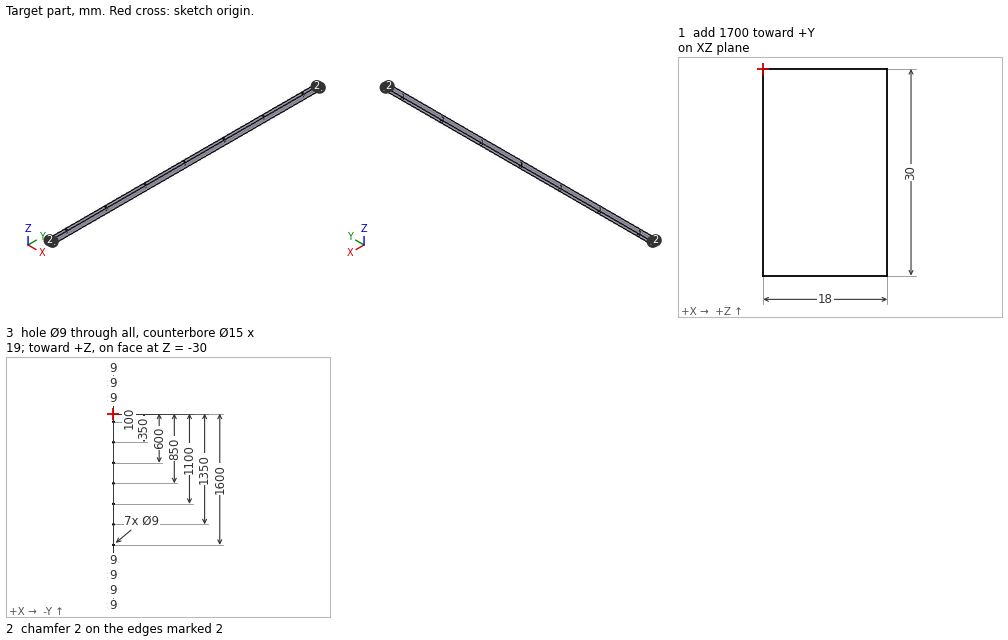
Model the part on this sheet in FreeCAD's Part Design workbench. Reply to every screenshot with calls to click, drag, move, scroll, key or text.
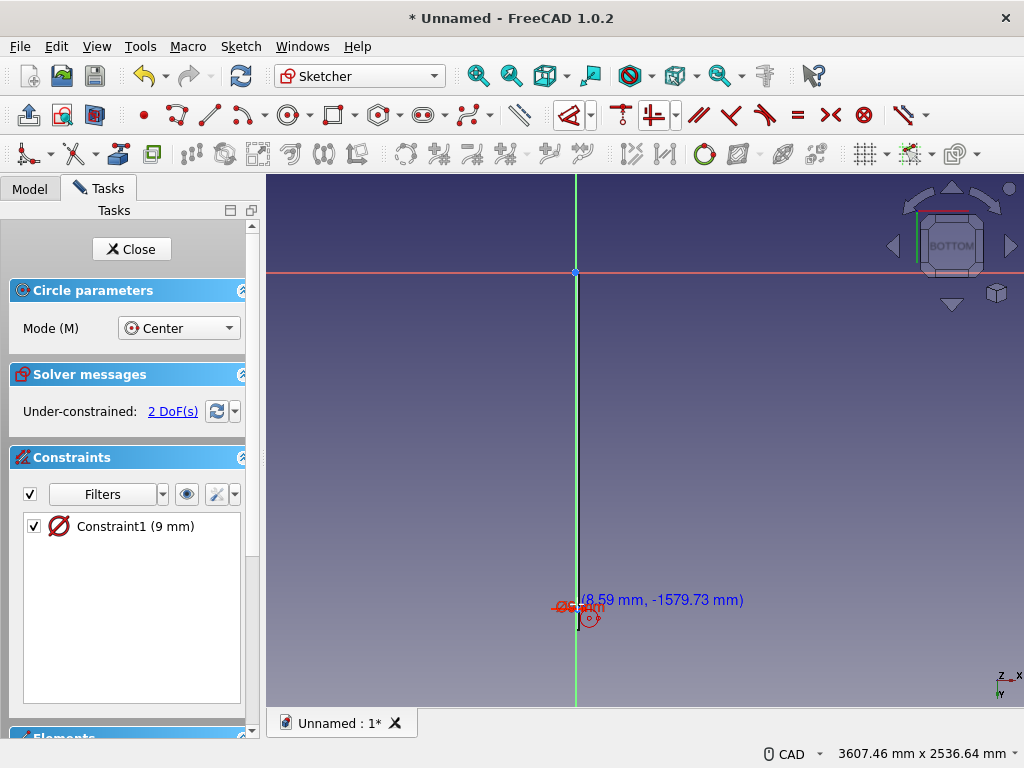
scroll(577, 557, up, 16)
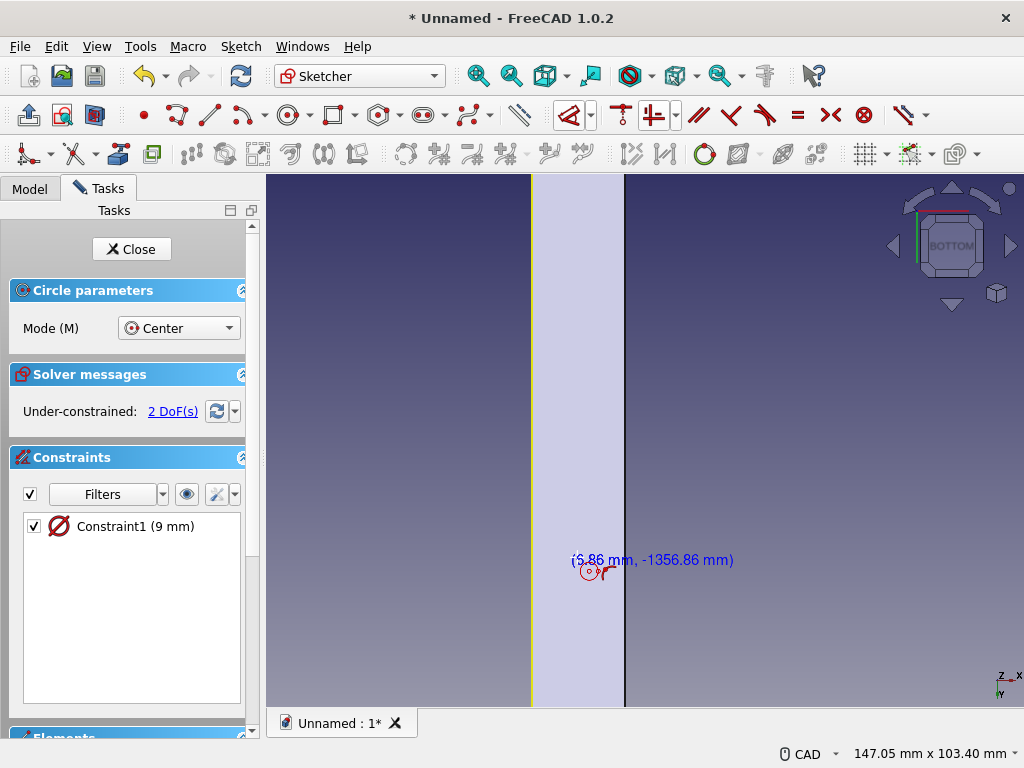
scroll(577, 584, down, 15)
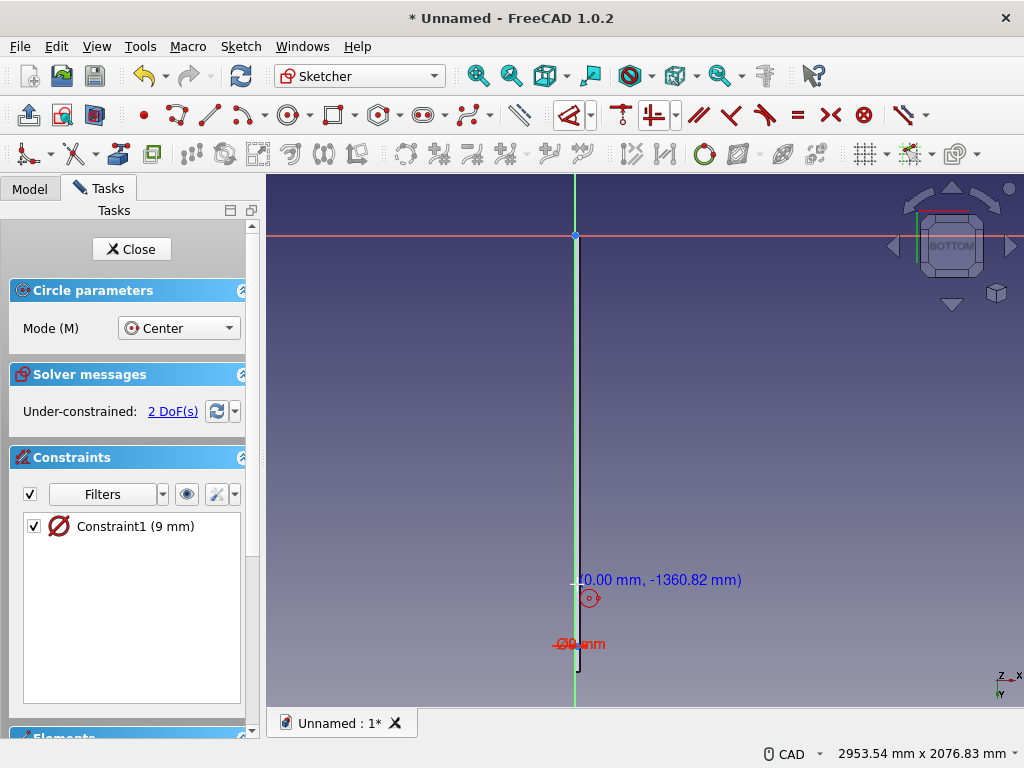
scroll(577, 582, up, 10)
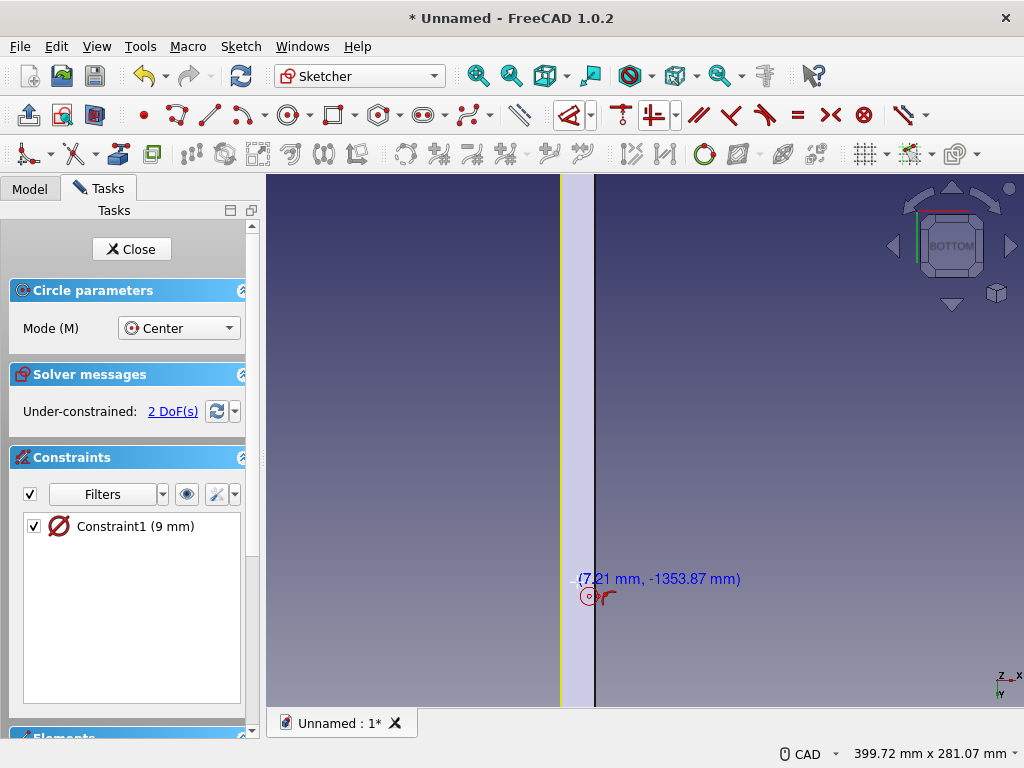
click(578, 577)
move(584, 571)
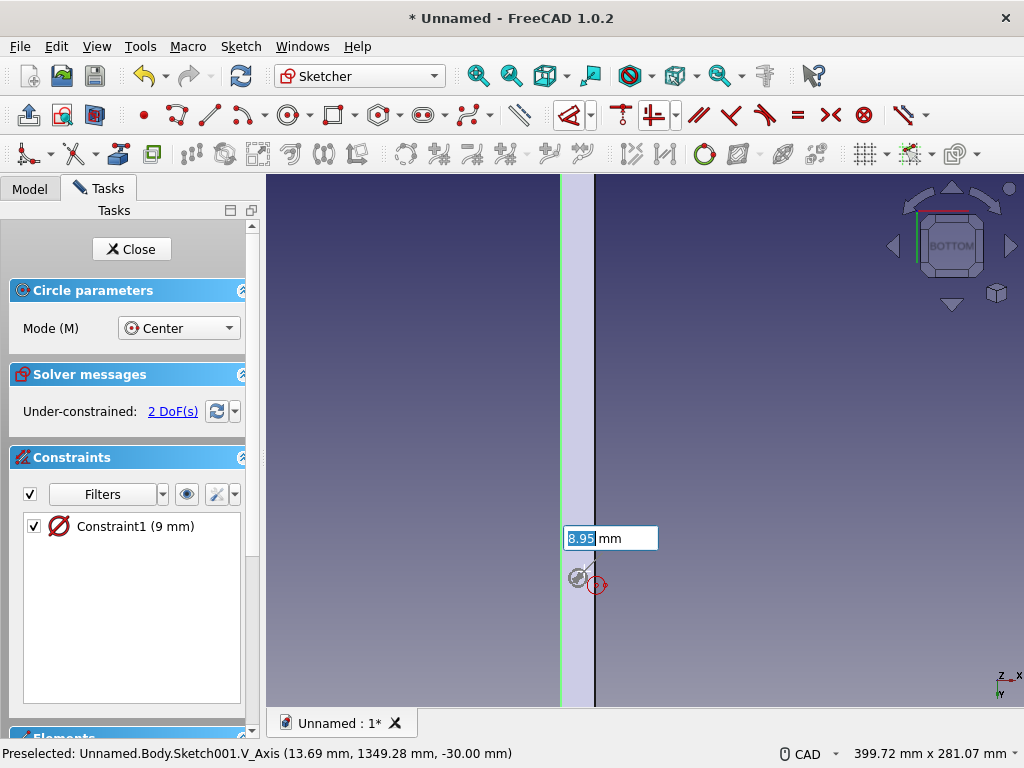
text(9)
key(Return)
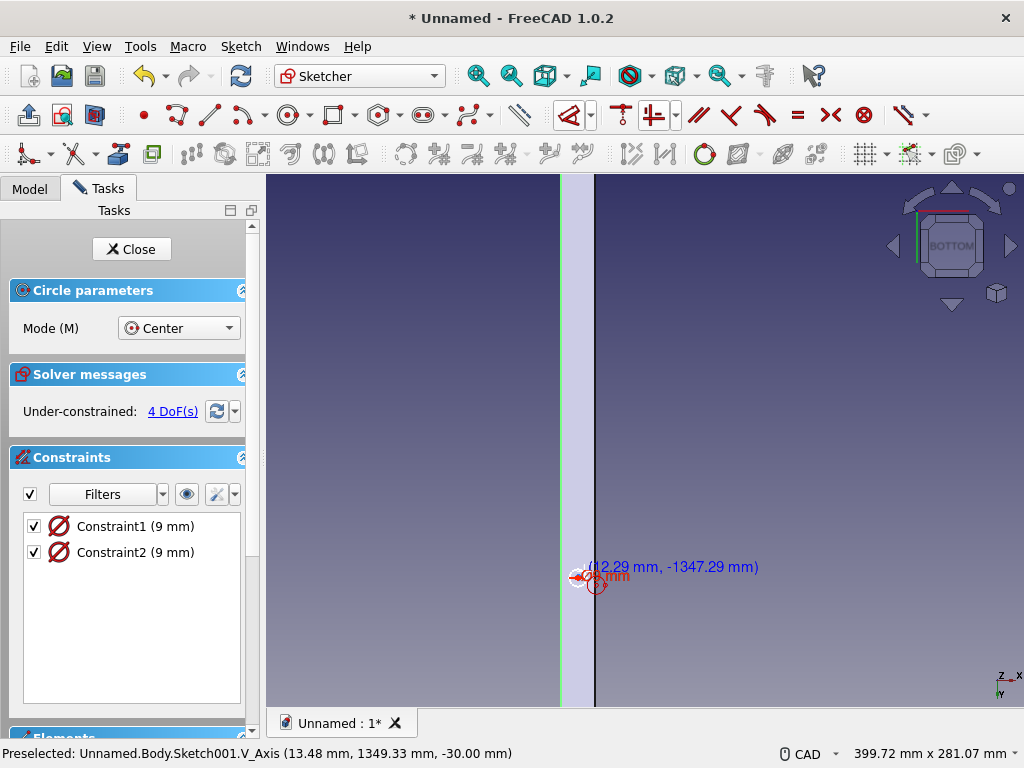
scroll(577, 553, down, 11)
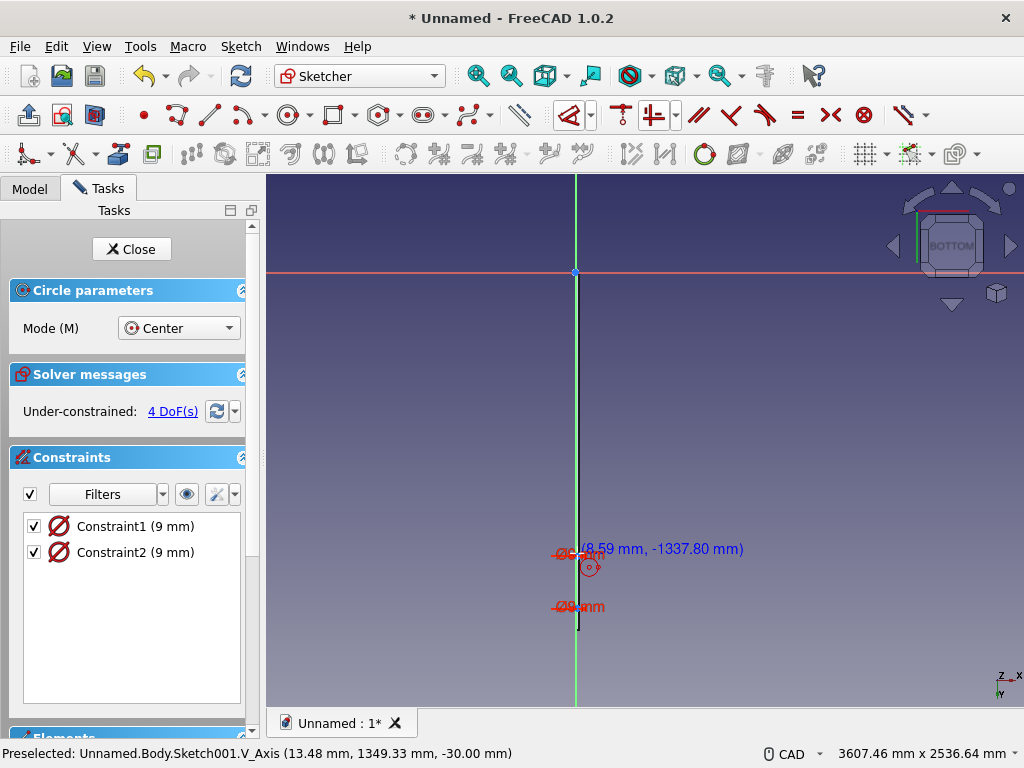
scroll(577, 504, up, 16)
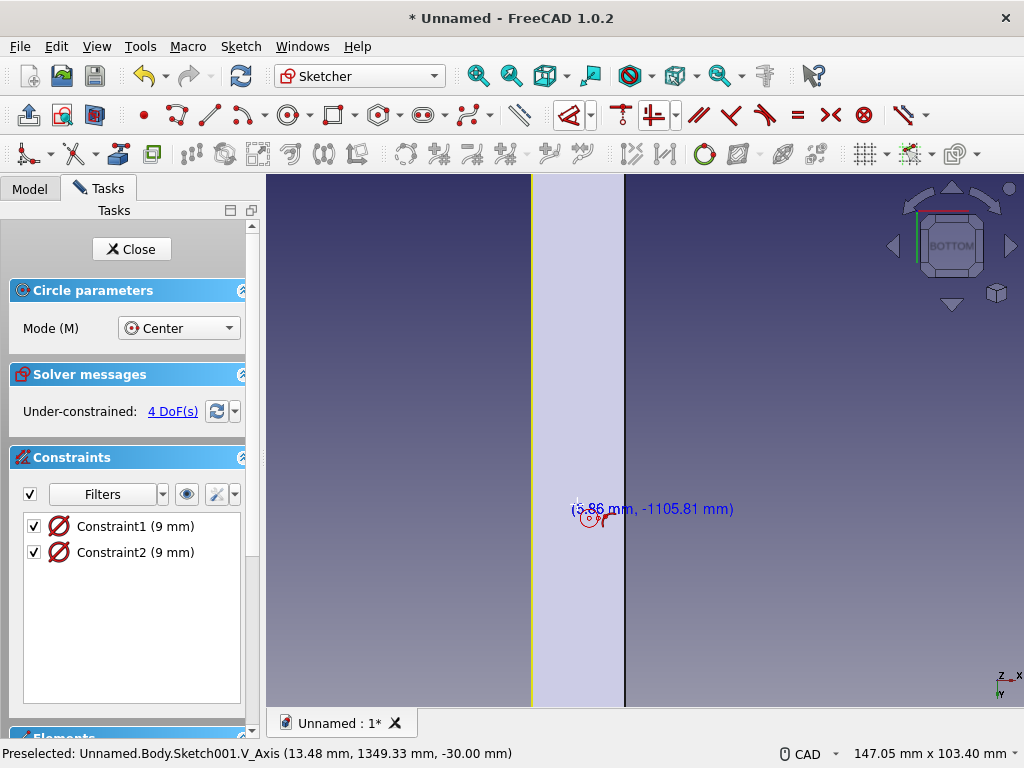
scroll(577, 519, down, 15)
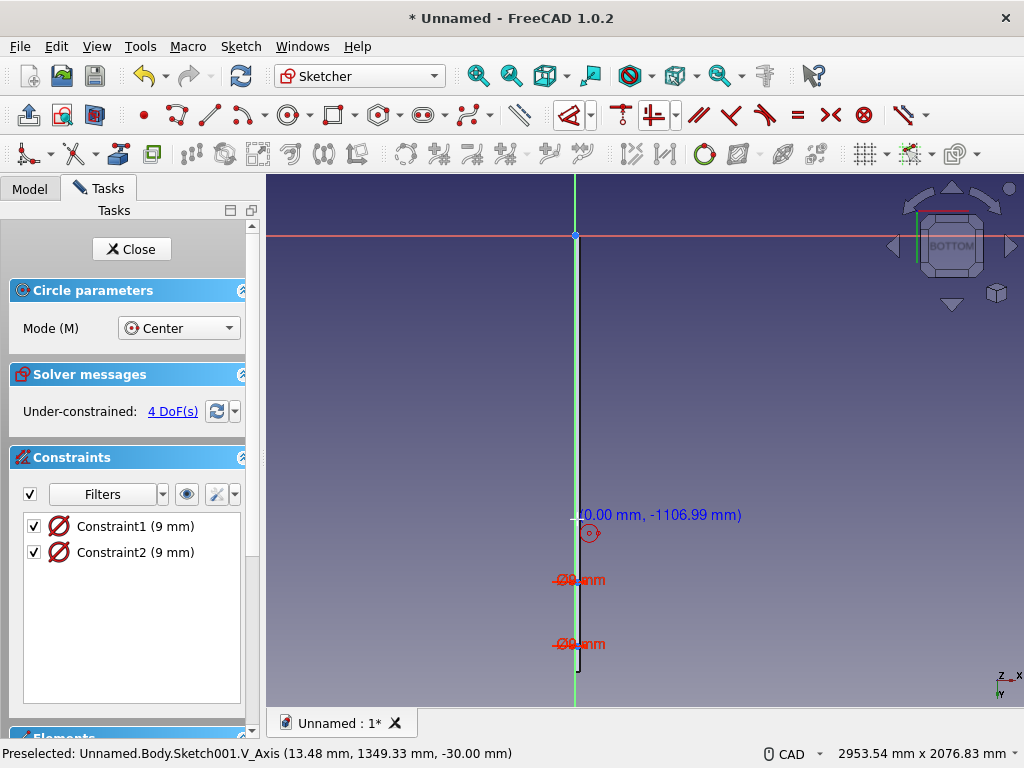
scroll(577, 518, up, 10)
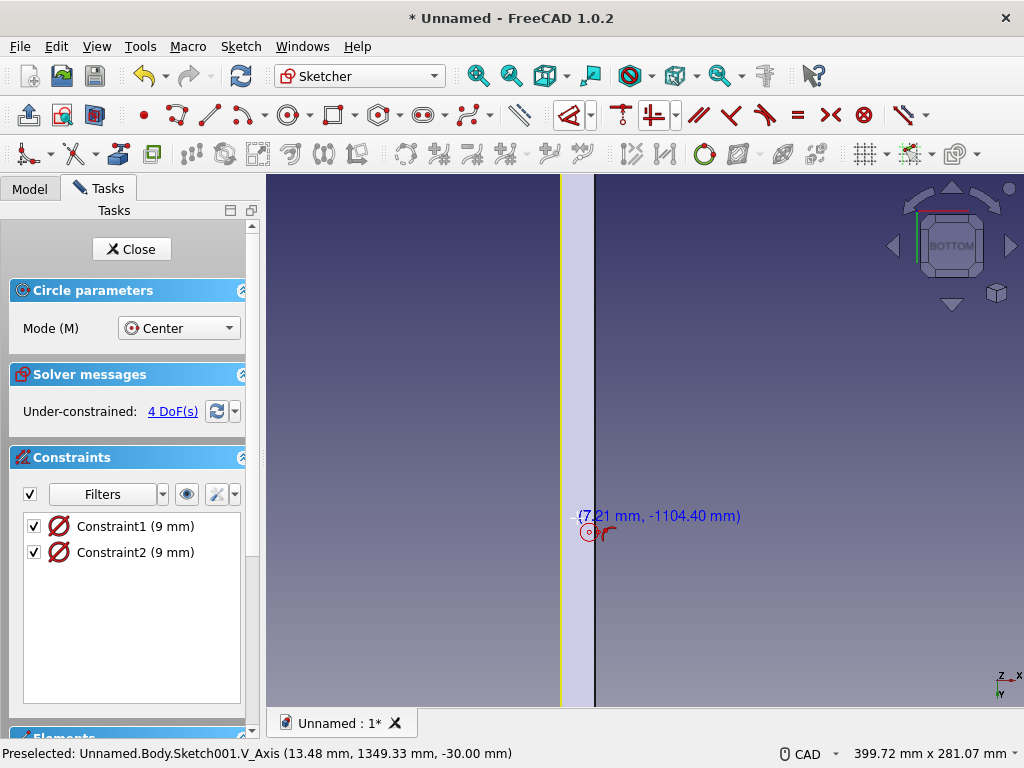
click(578, 513)
move(584, 507)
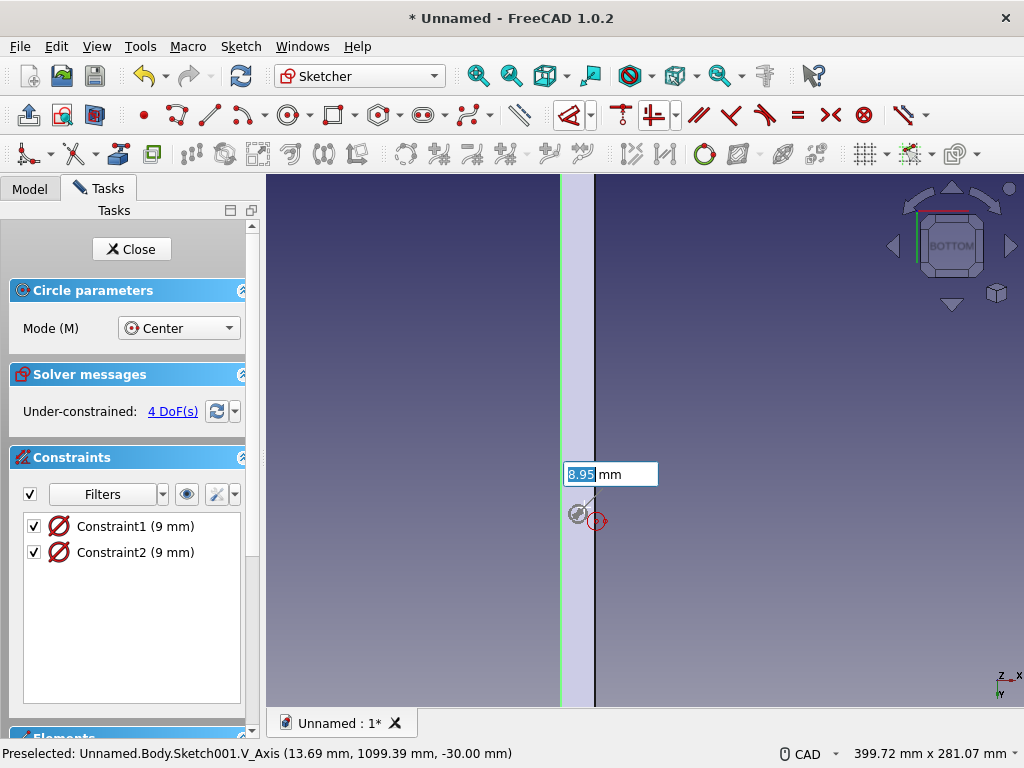
text(9)
key(Return)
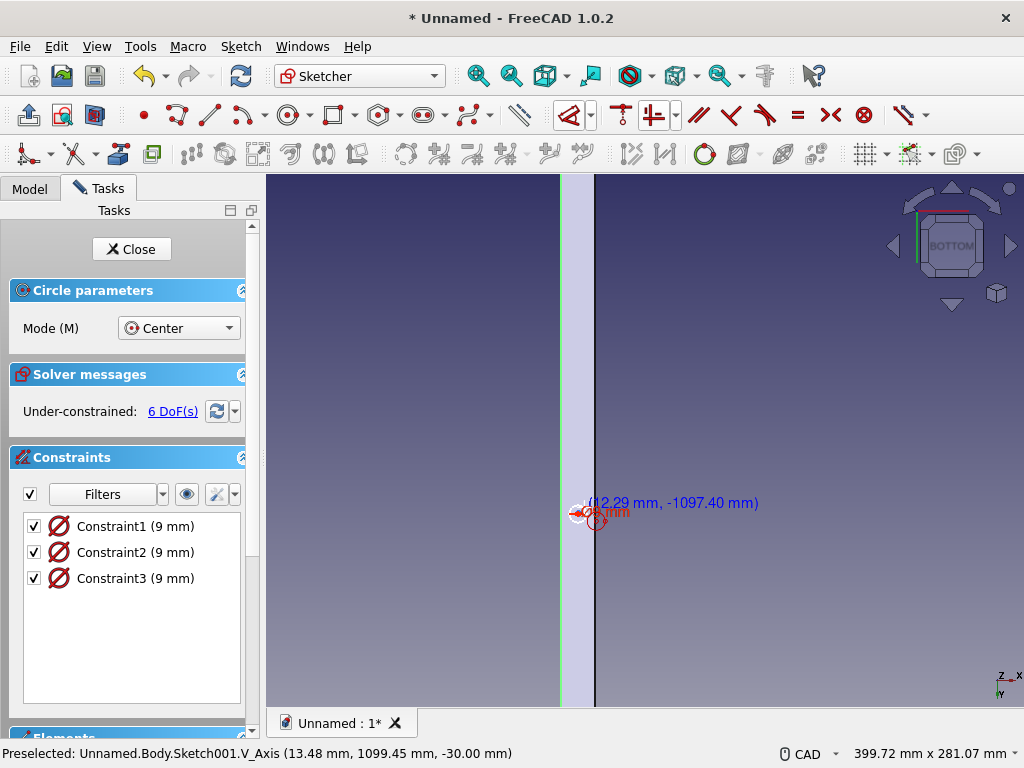
scroll(577, 502, down, 11)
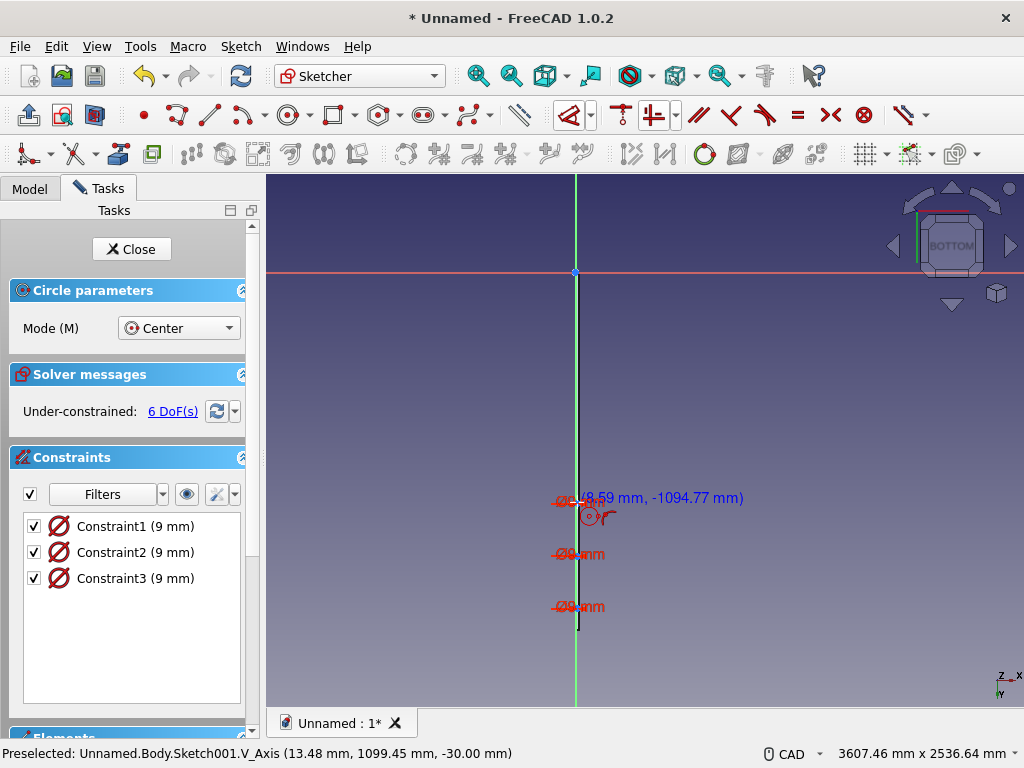
scroll(577, 399, up, 16)